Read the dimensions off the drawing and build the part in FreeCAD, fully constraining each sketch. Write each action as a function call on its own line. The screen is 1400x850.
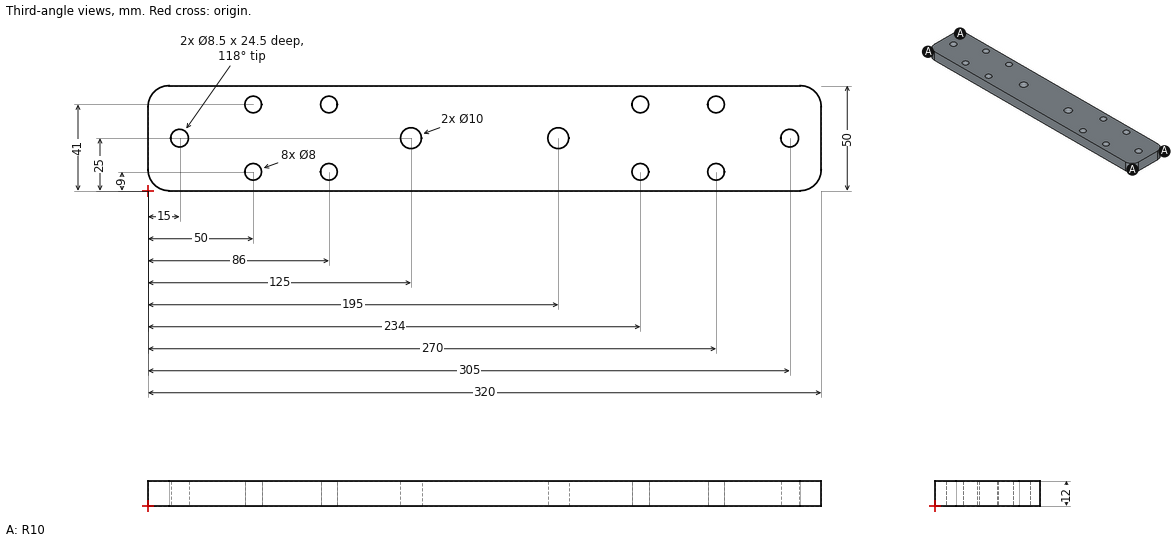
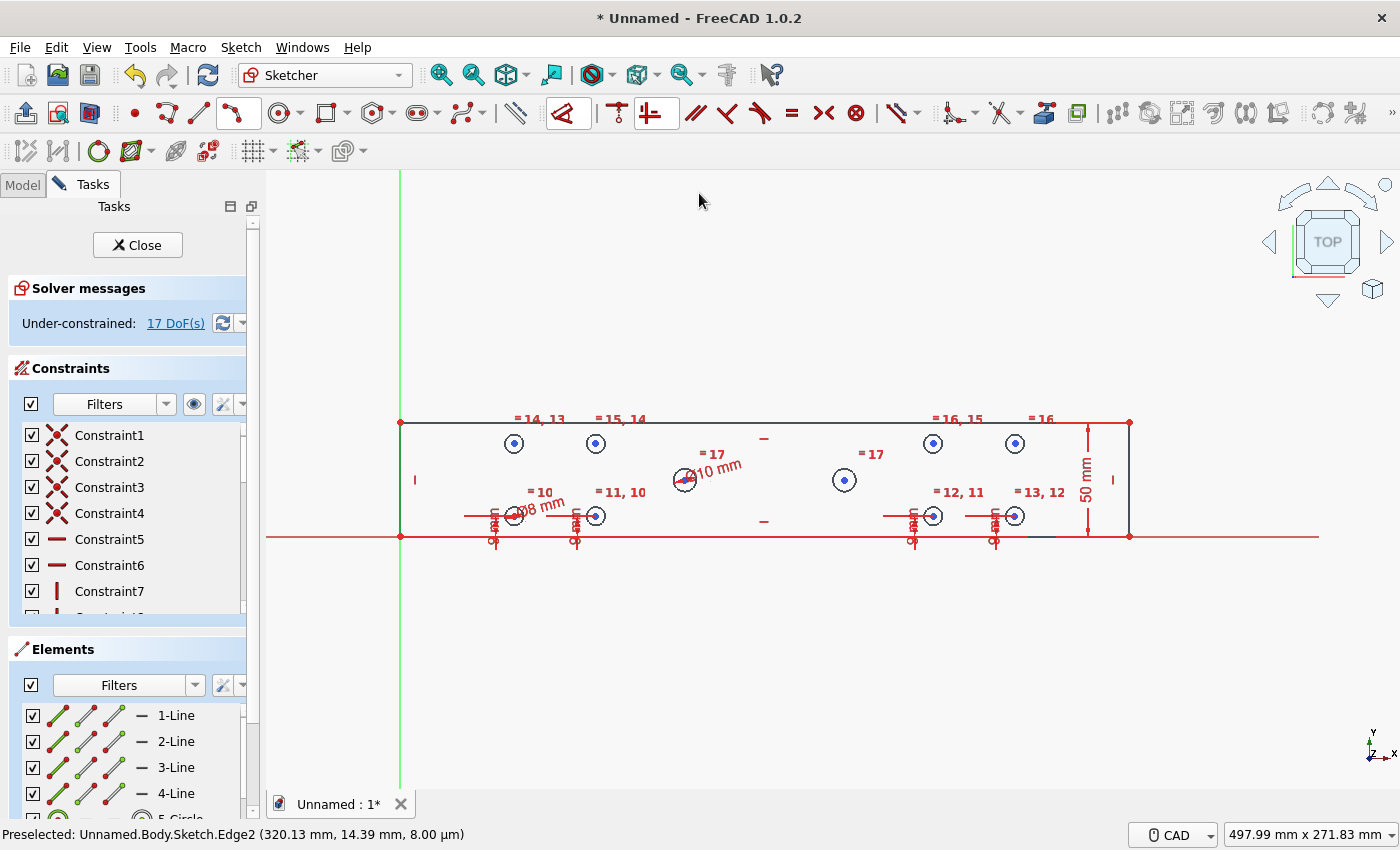
click(514, 516)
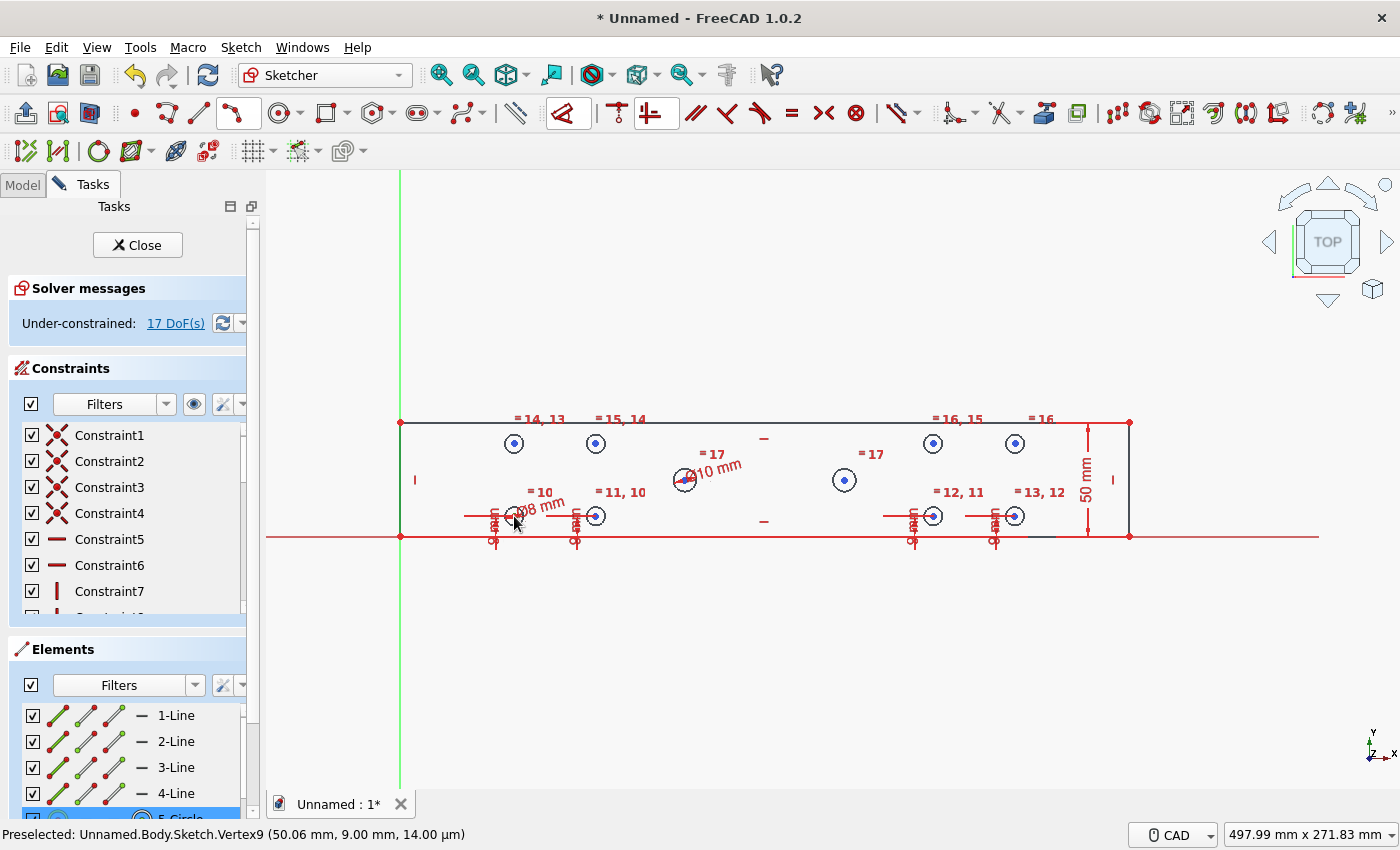
key(l)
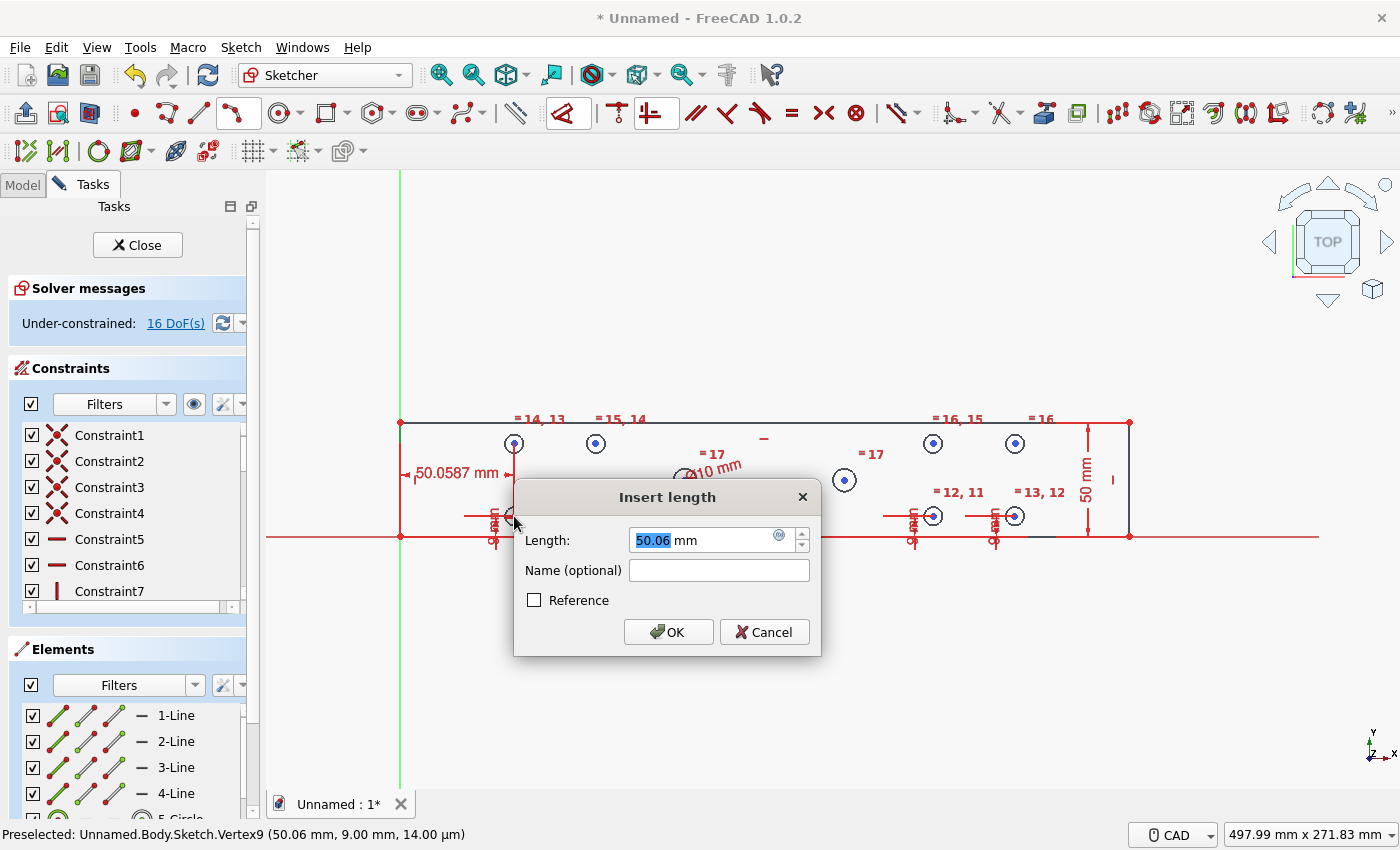
text(50)
key(Return)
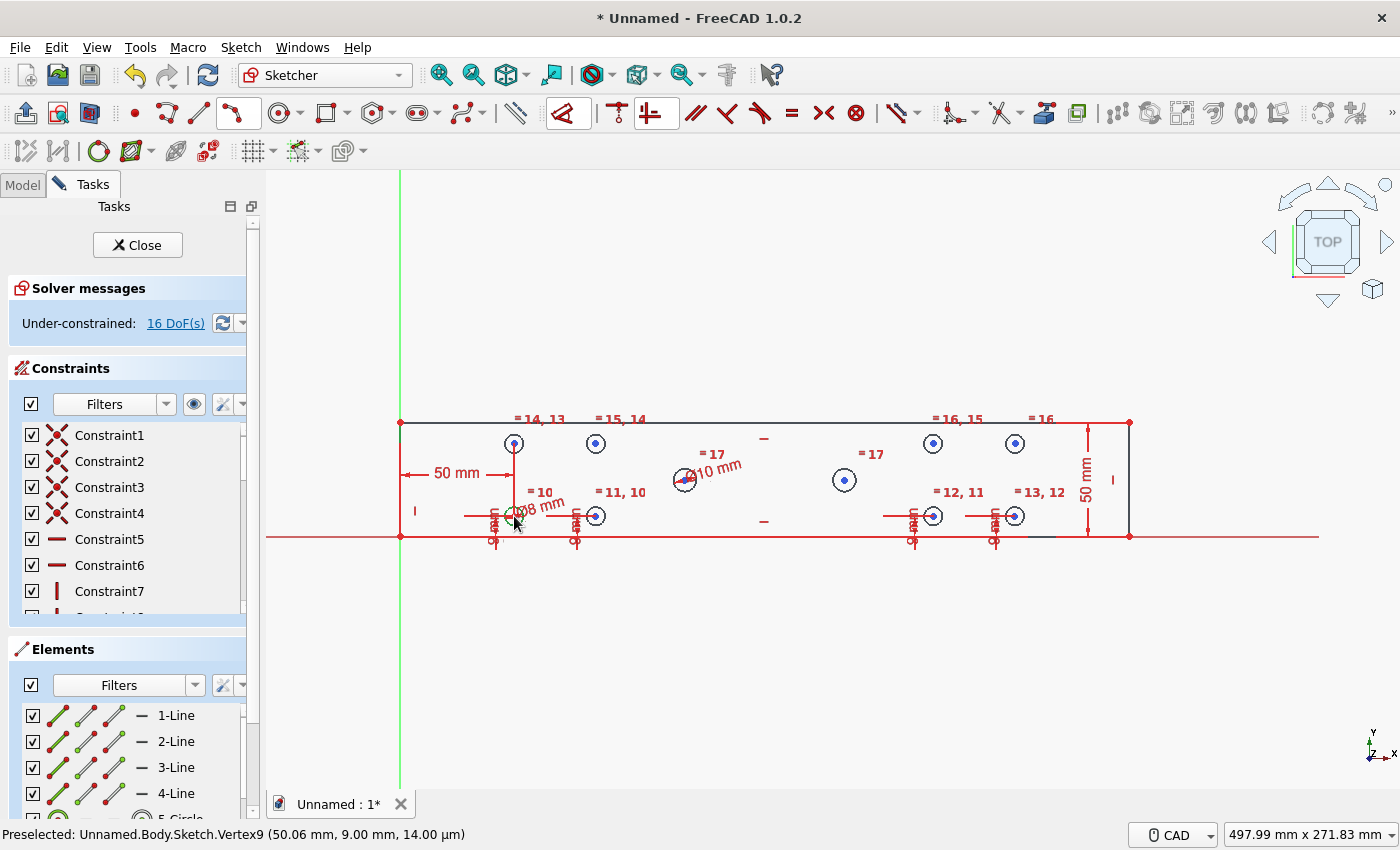
click(596, 516)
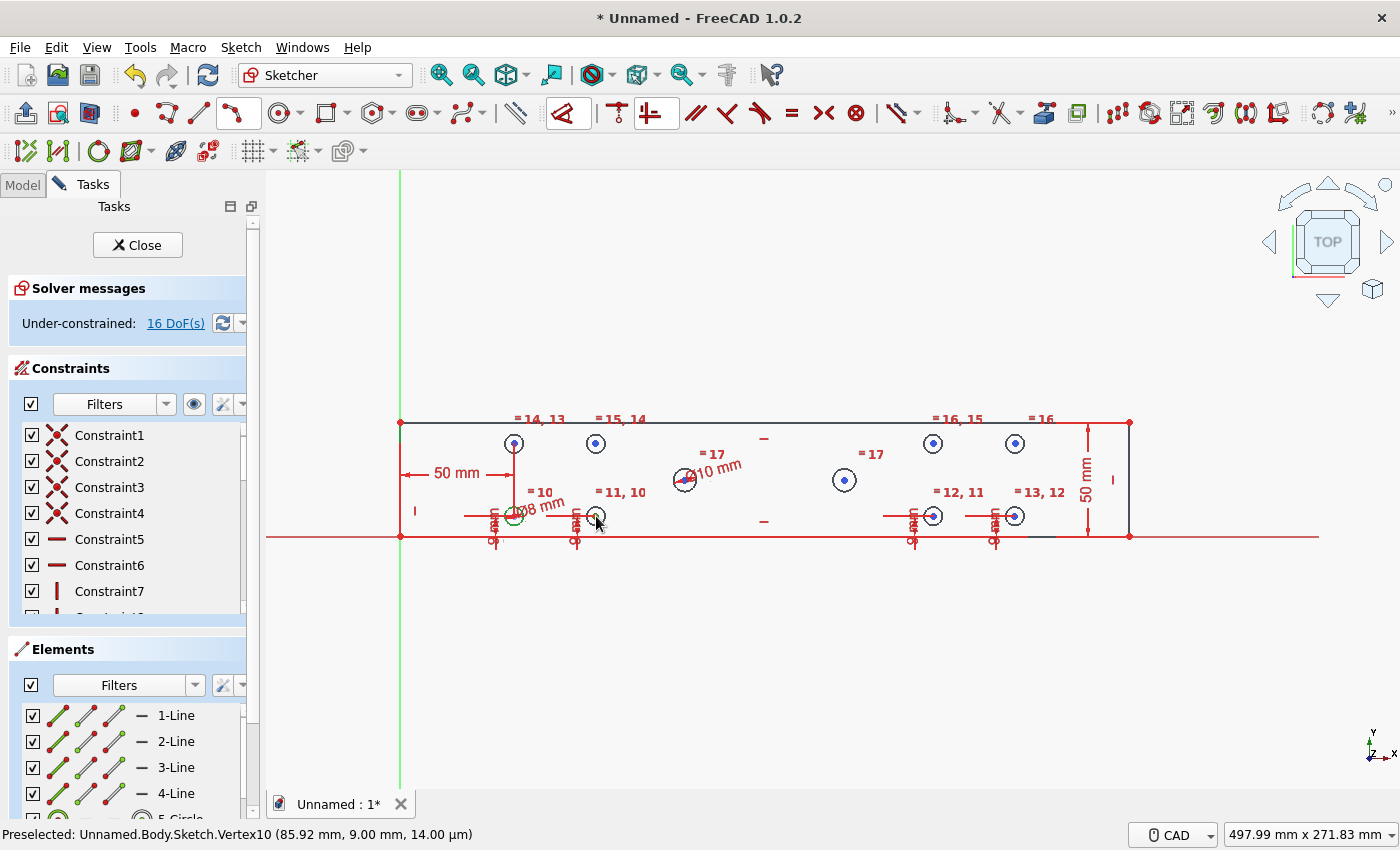
key(l)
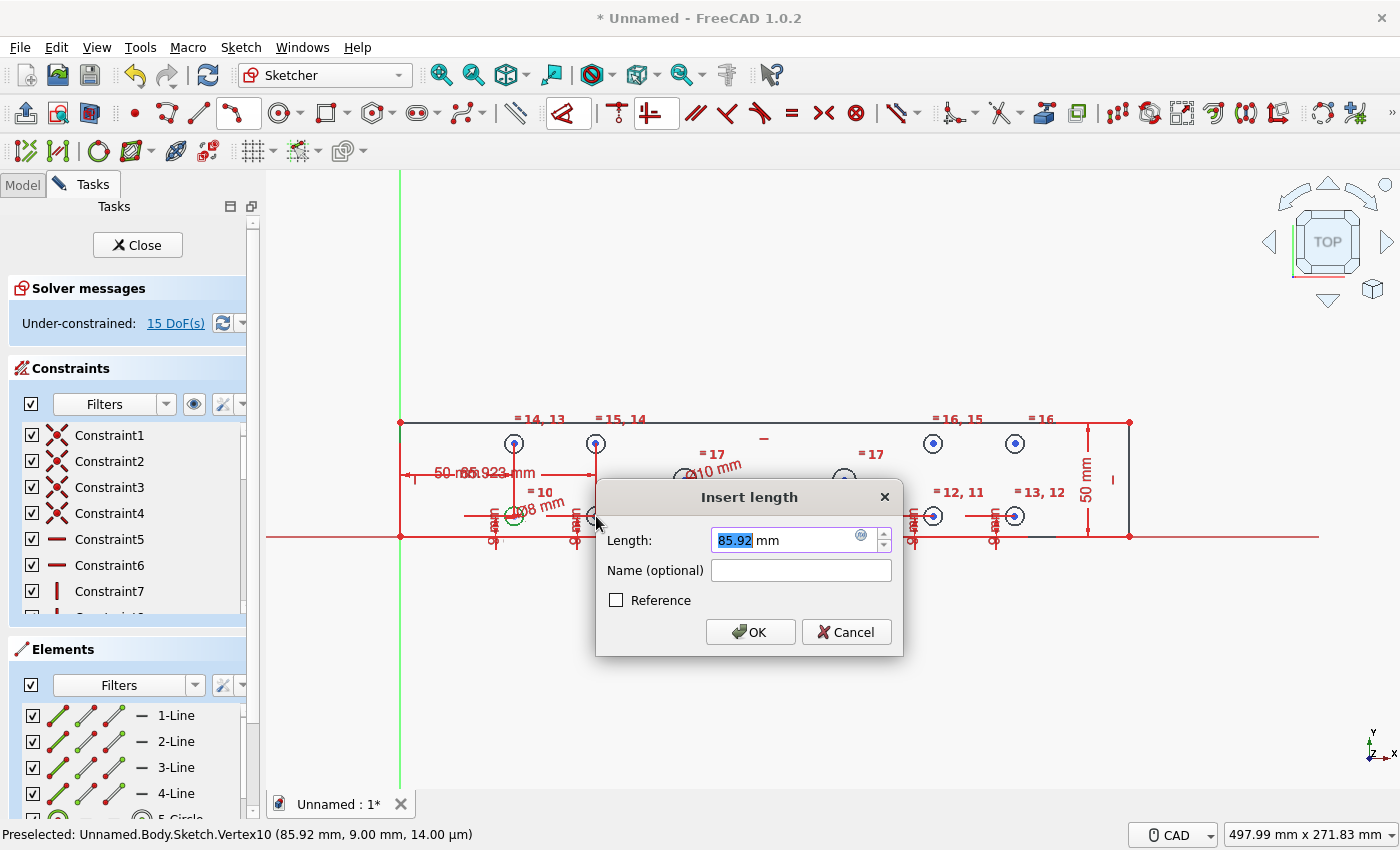
text(86)
key(Return)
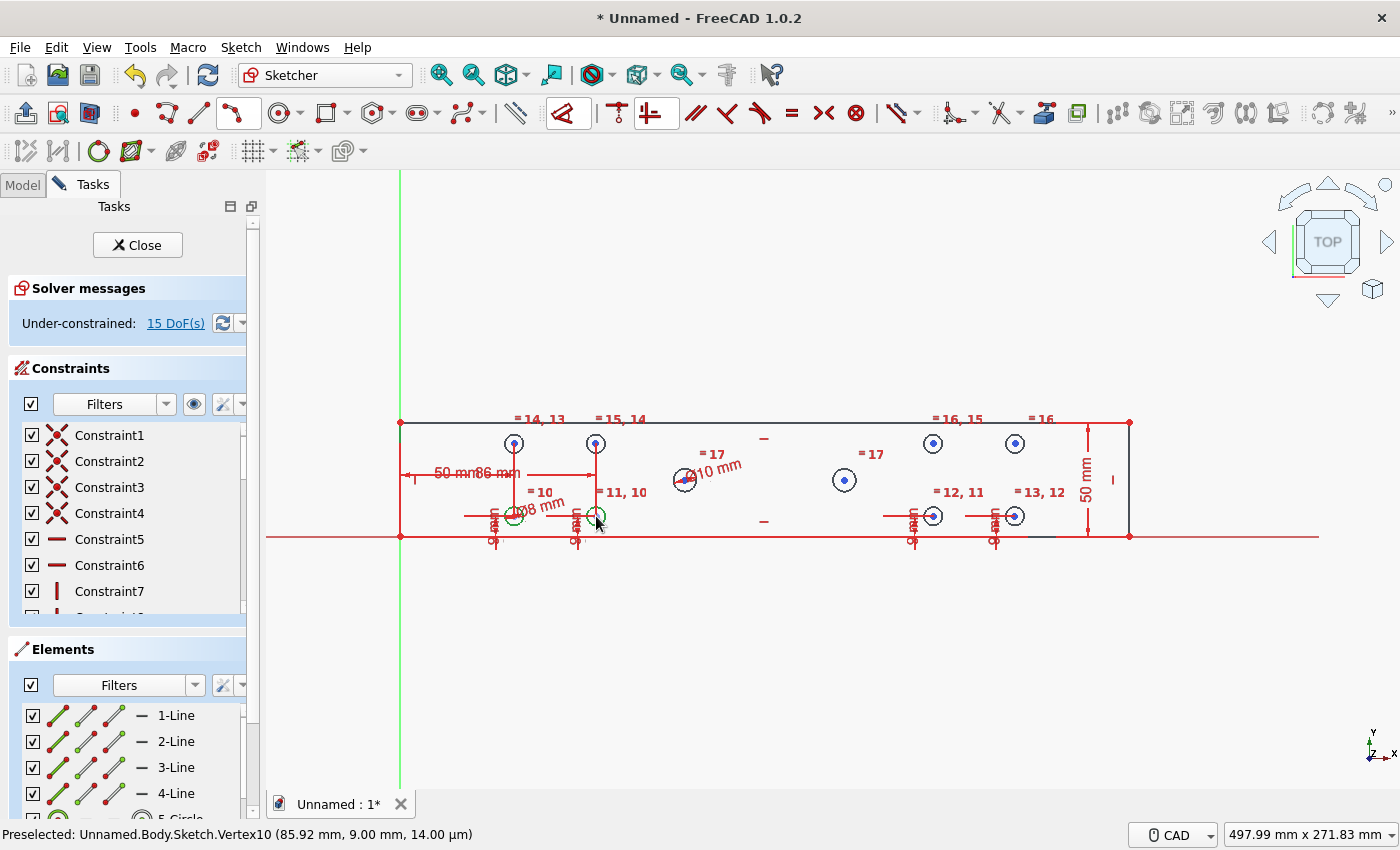
click(685, 480)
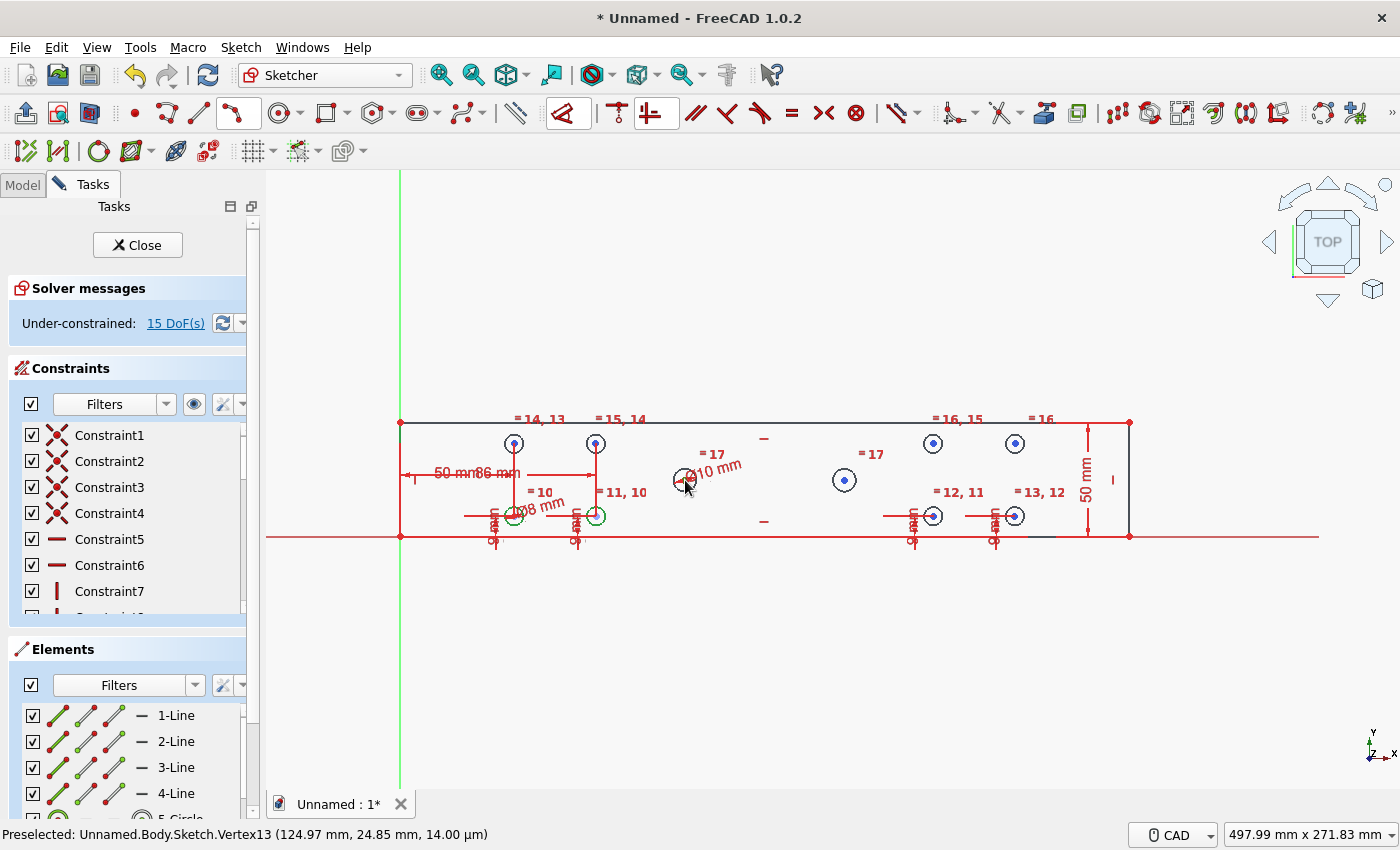
key(i)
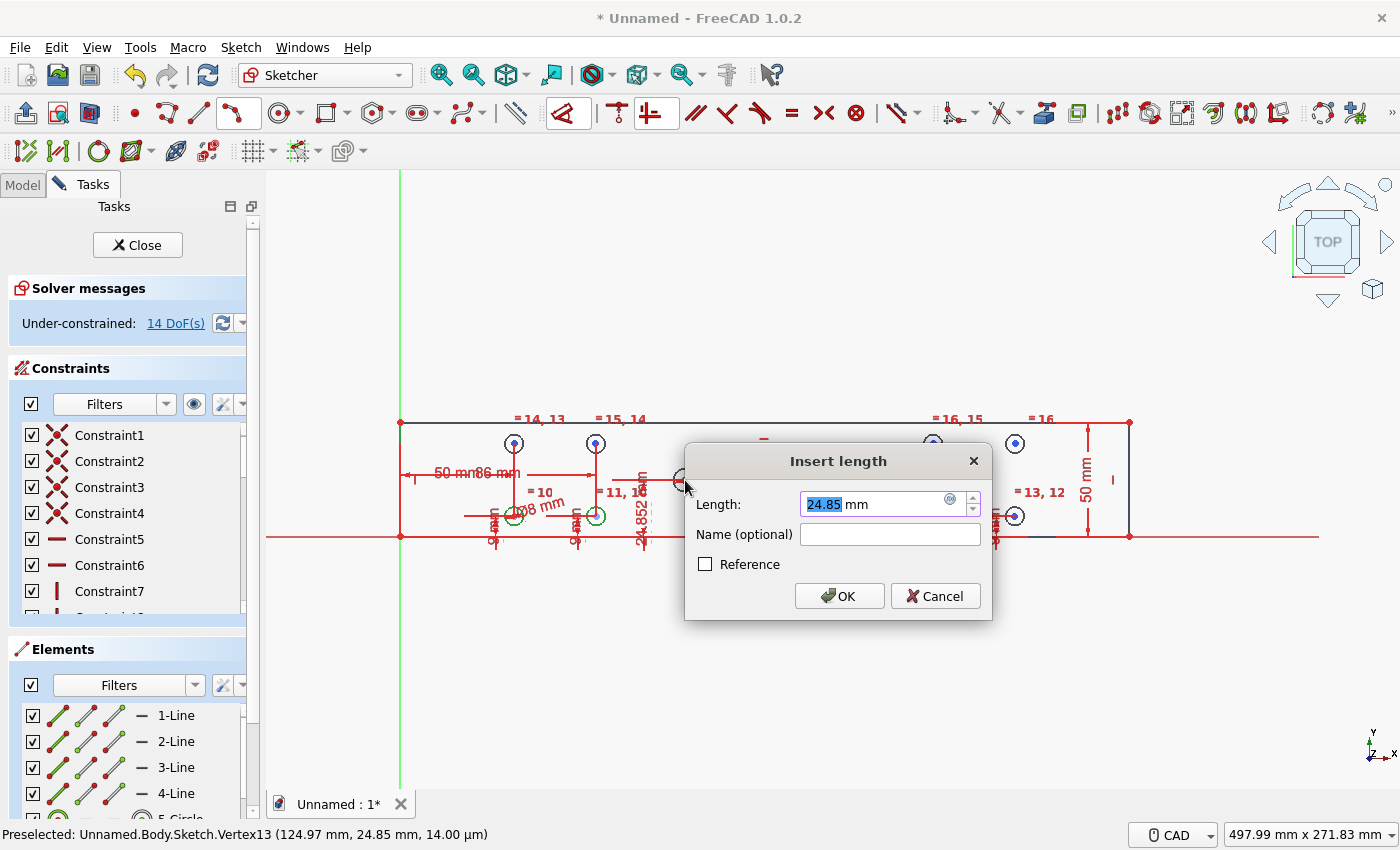
text(25)
key(Return)